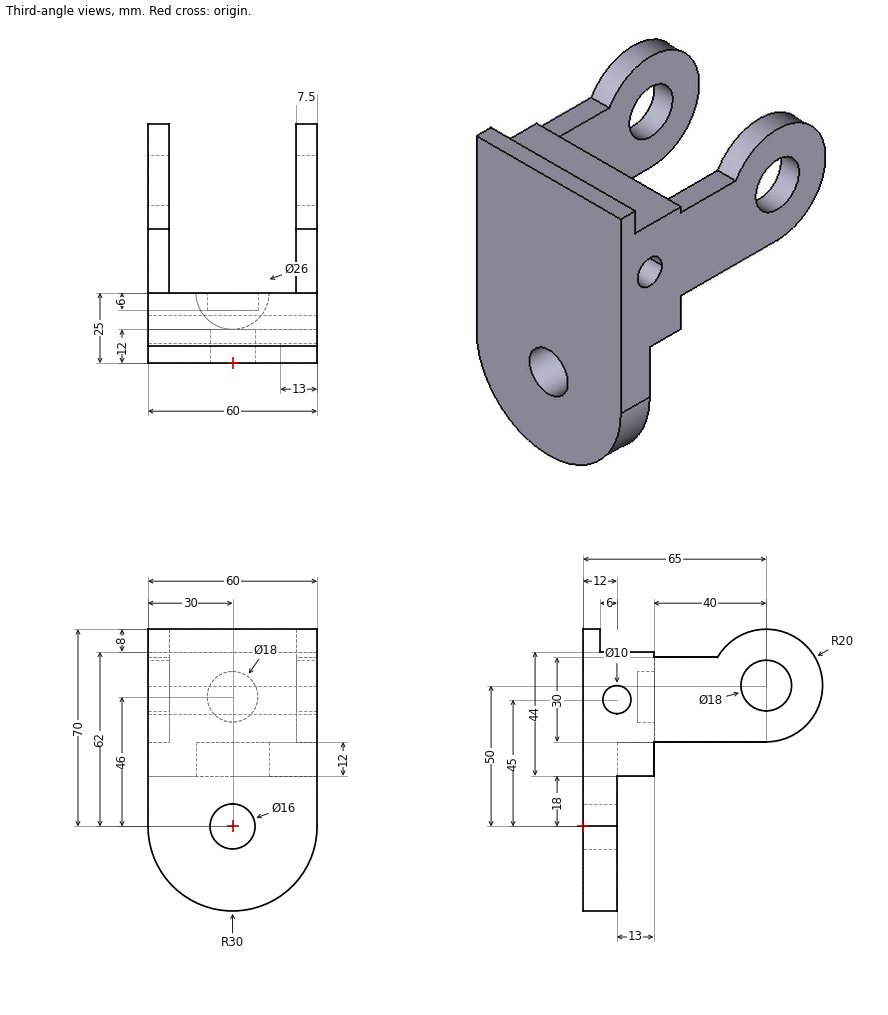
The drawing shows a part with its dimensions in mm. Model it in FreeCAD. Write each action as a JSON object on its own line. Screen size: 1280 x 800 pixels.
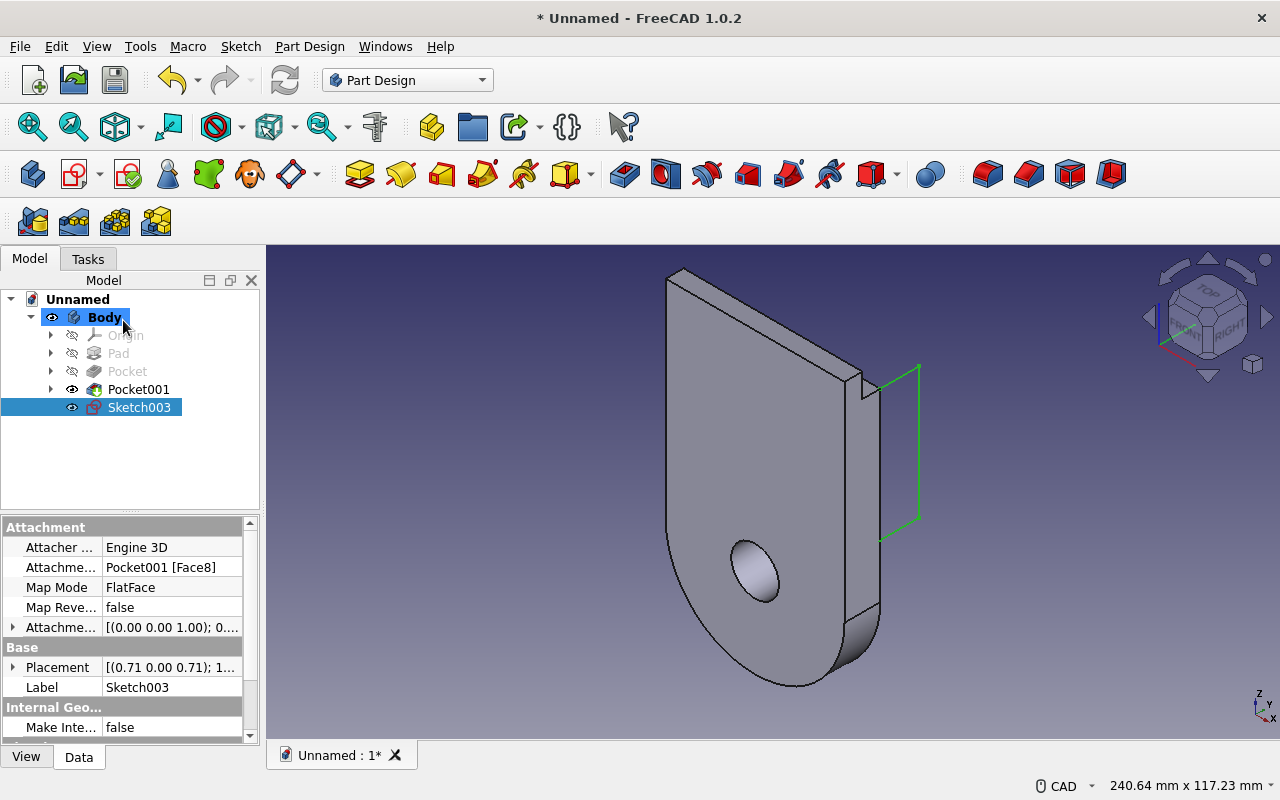
{"action": "left_click", "coordinate": [360, 174]}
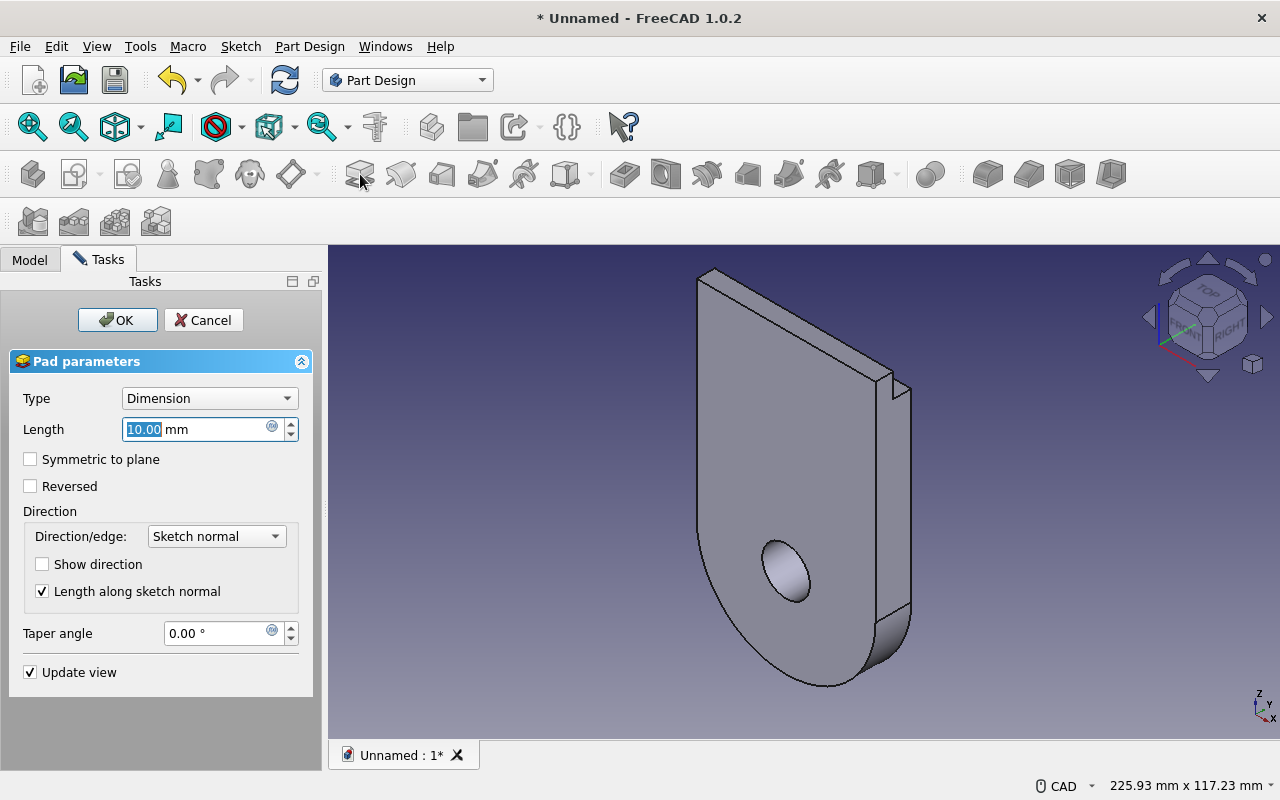
{"action": "type", "text": "60"}
{"action": "key", "text": "Tab"}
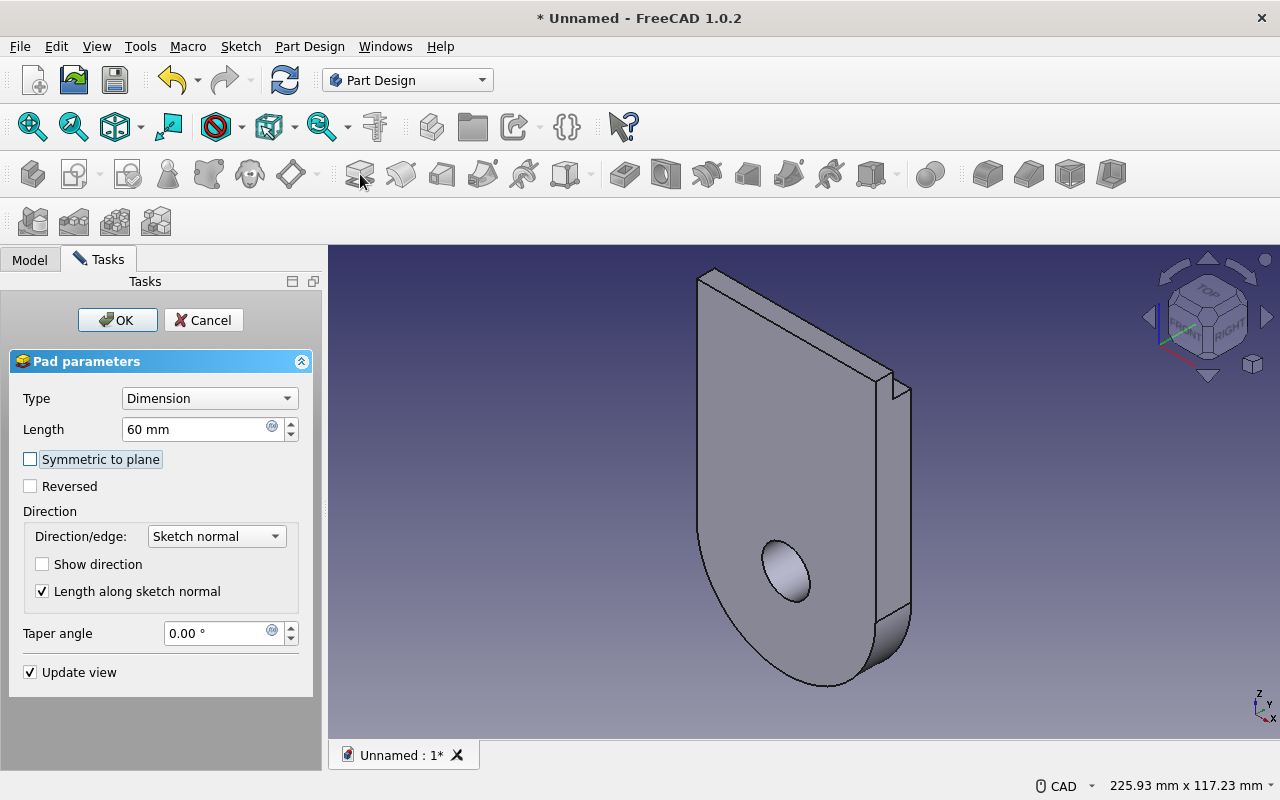
{"action": "left_click", "coordinate": [31, 486]}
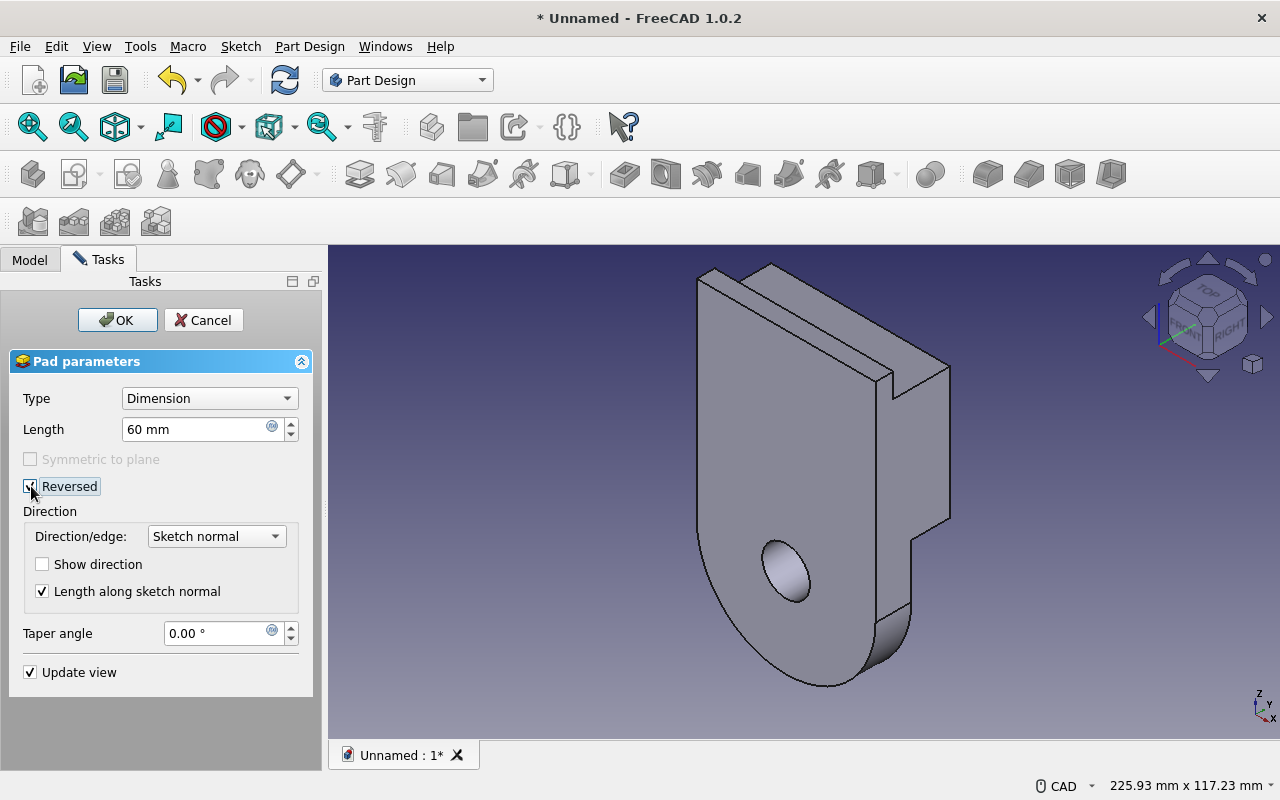
{"action": "left_click", "coordinate": [118, 320]}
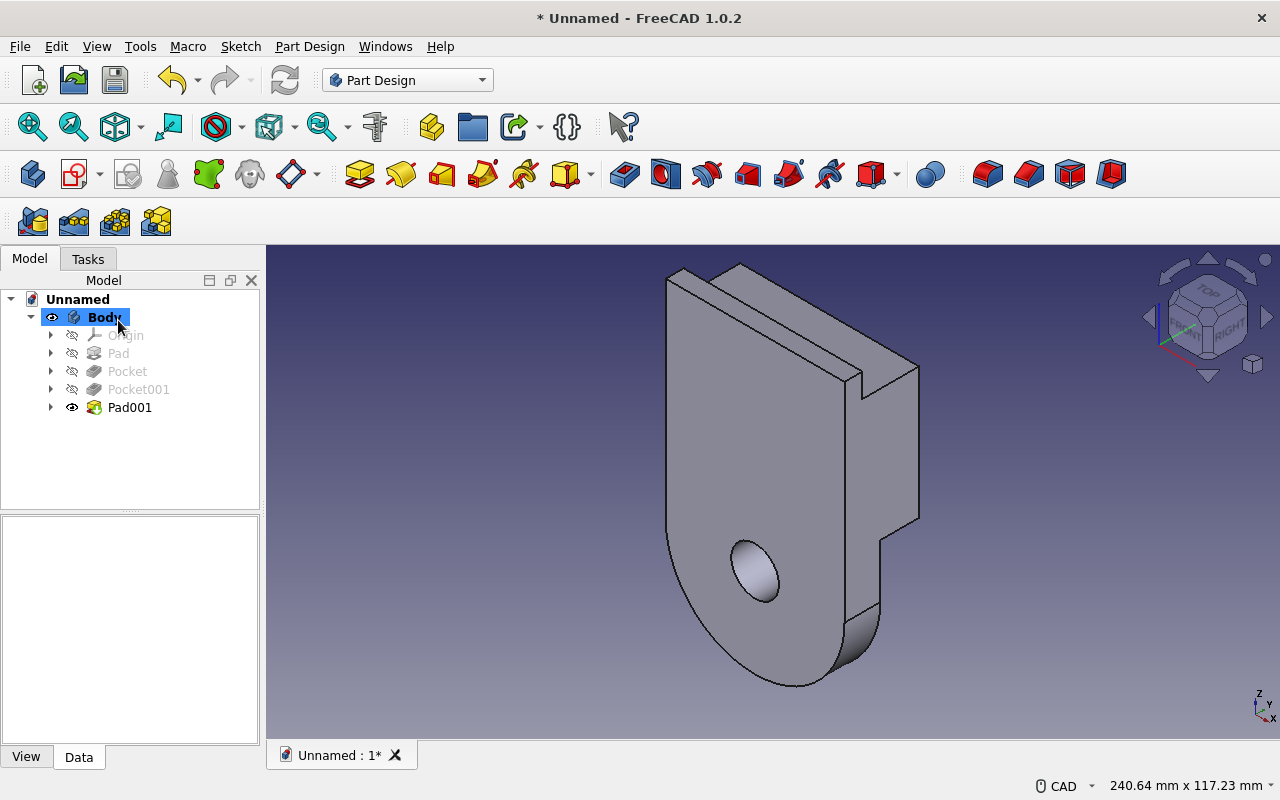
{"action": "key", "text": "v f"}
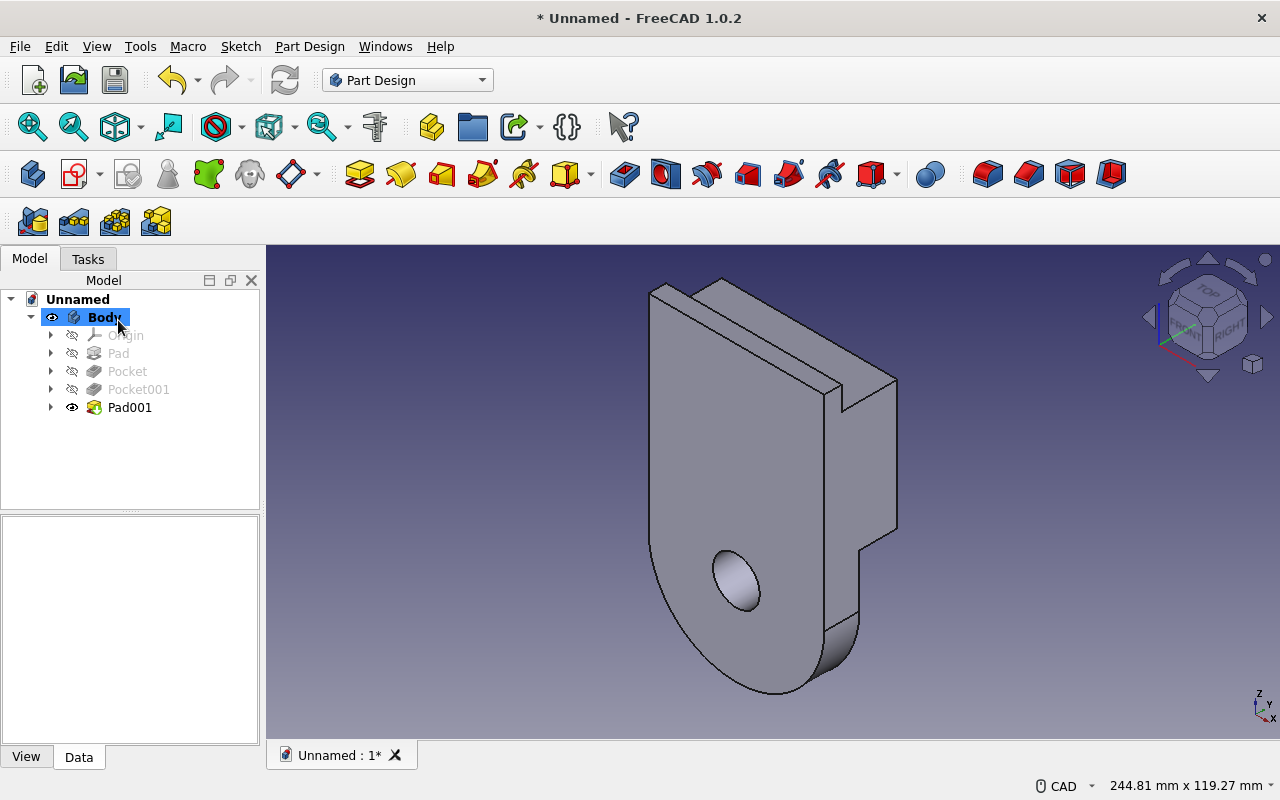
{"action": "left_click", "coordinate": [861, 491]}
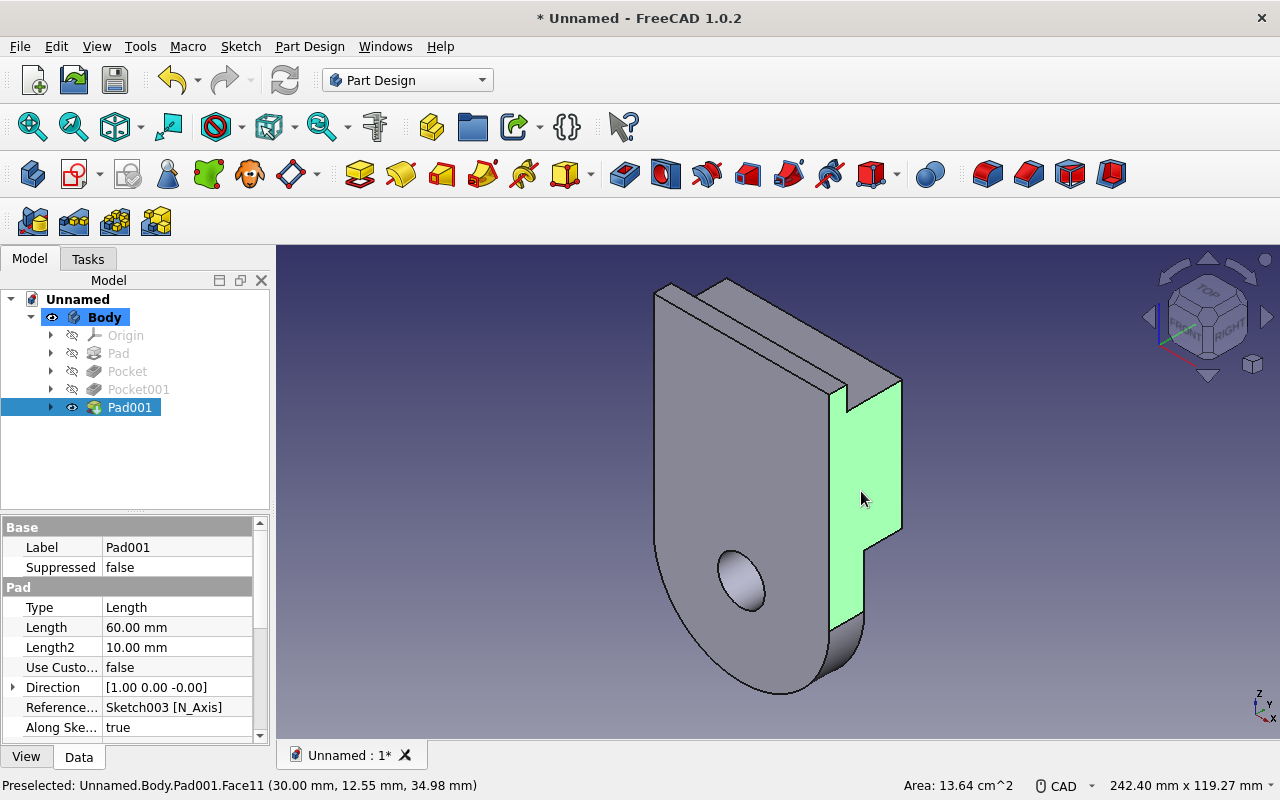
{"action": "left_click", "coordinate": [74, 174]}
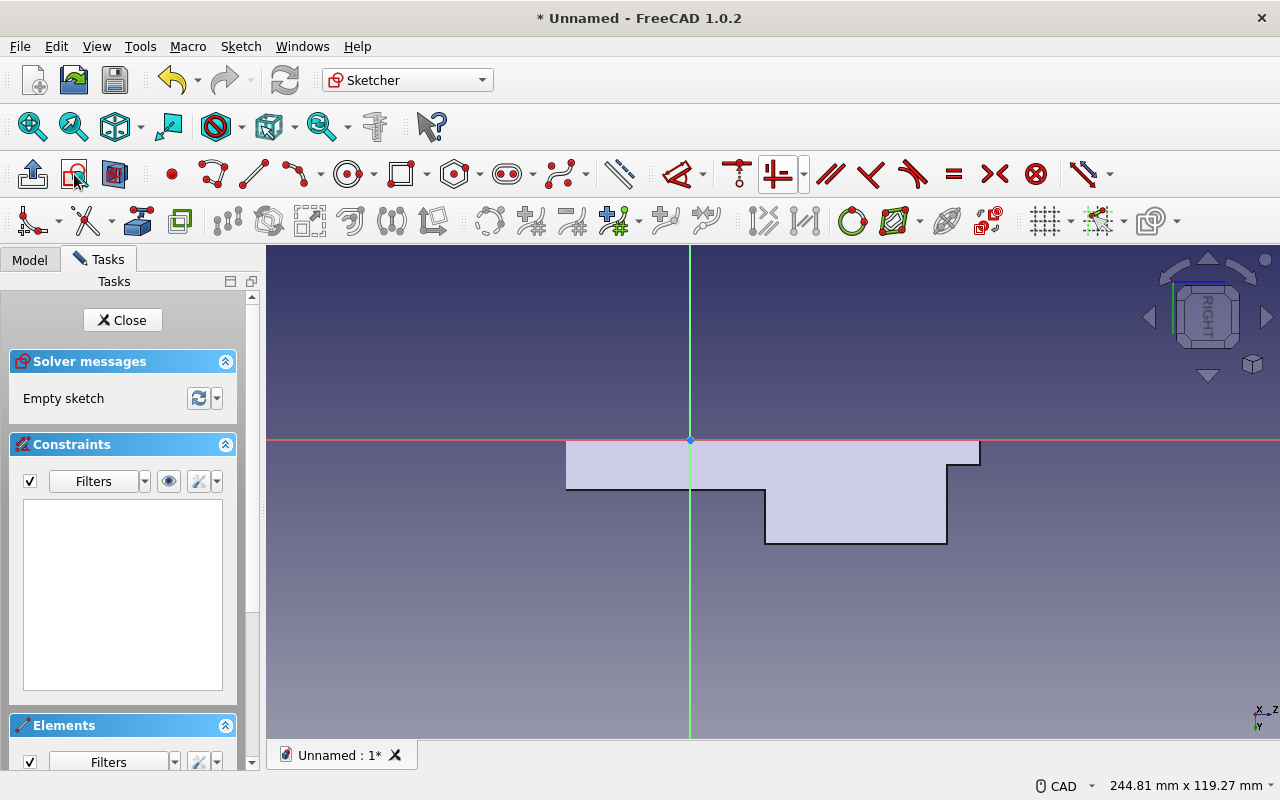
{"action": "scroll", "coordinate": [481, 273], "scroll_direction": "down", "scroll_amount": 2}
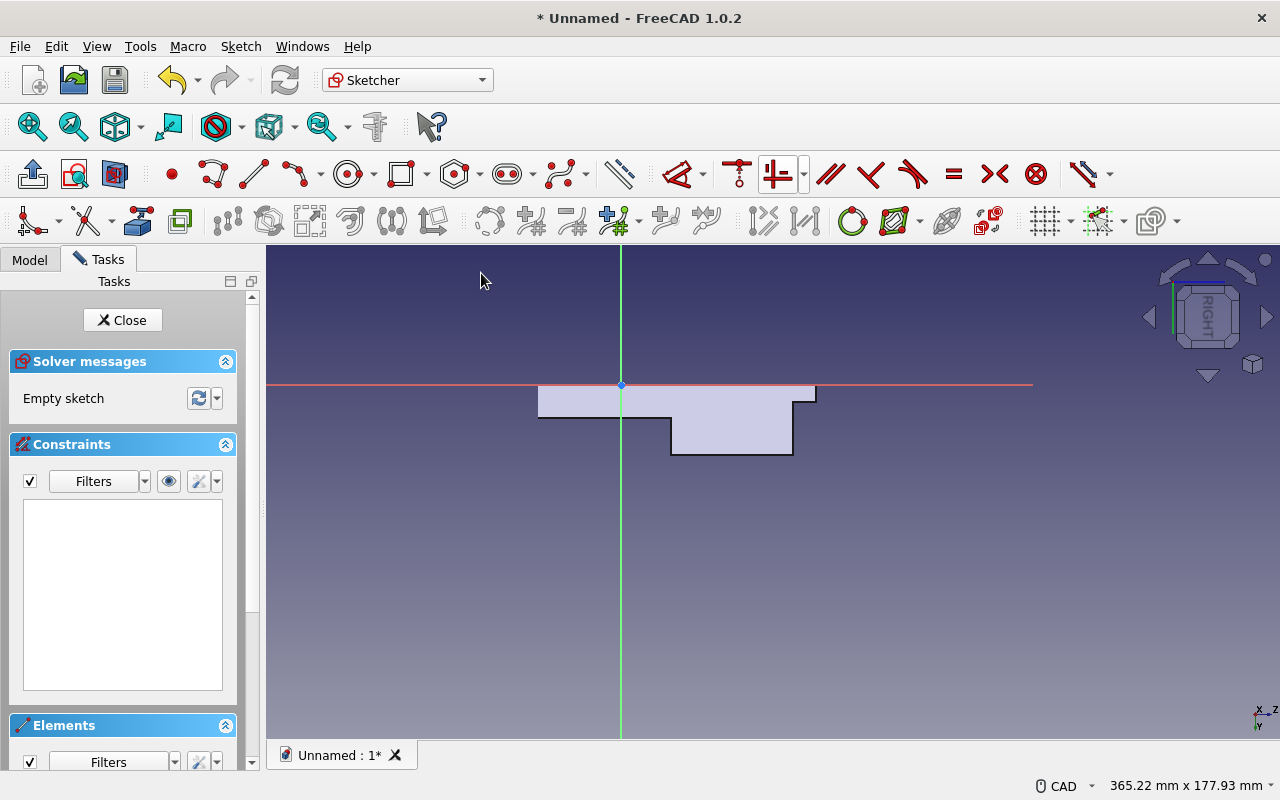
{"action": "scroll", "coordinate": [705, 514], "scroll_direction": "up", "scroll_amount": 2}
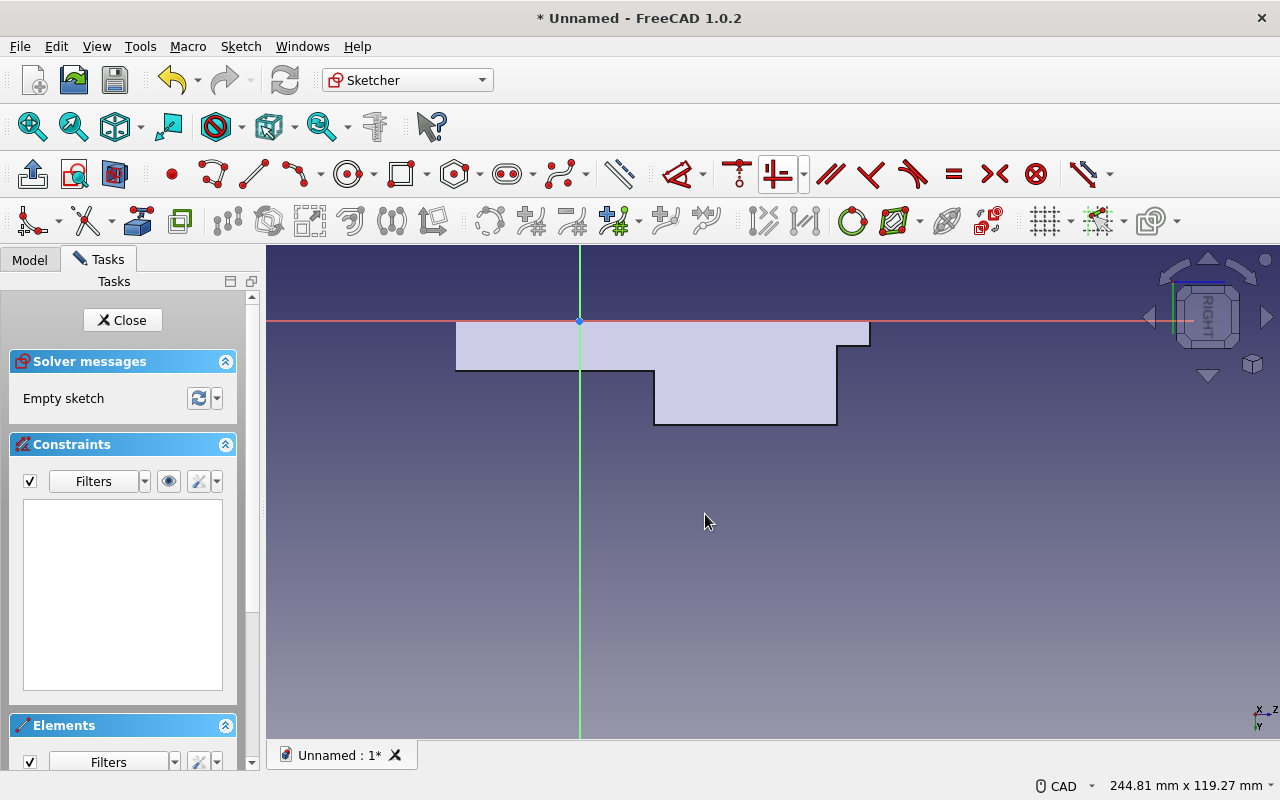
{"action": "key", "text": "g m"}